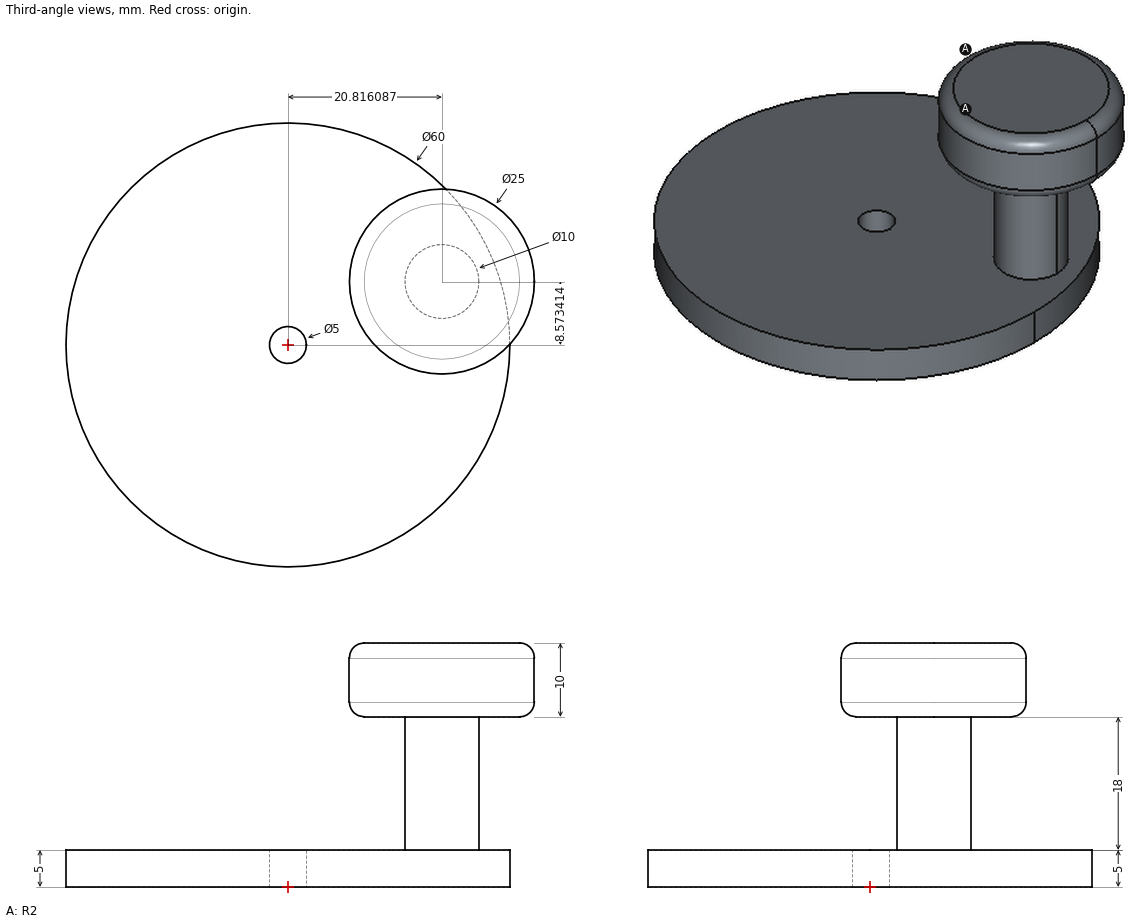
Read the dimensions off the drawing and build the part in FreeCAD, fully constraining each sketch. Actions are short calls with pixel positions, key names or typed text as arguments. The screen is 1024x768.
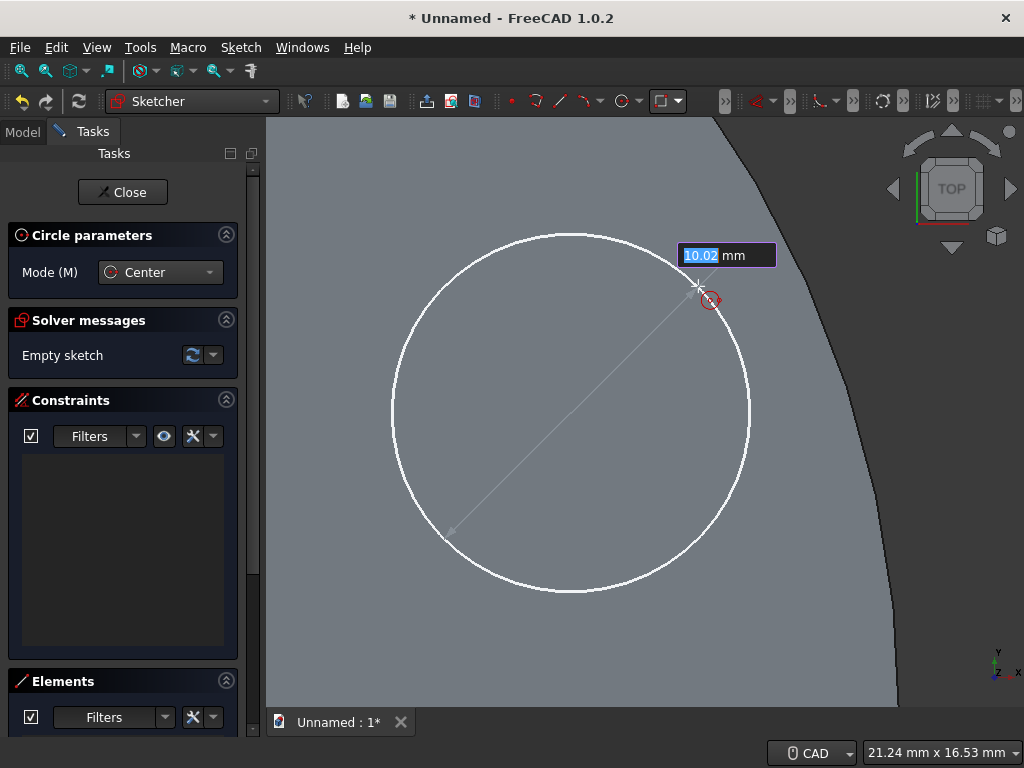
text(10)
key(Return)
key(Escape)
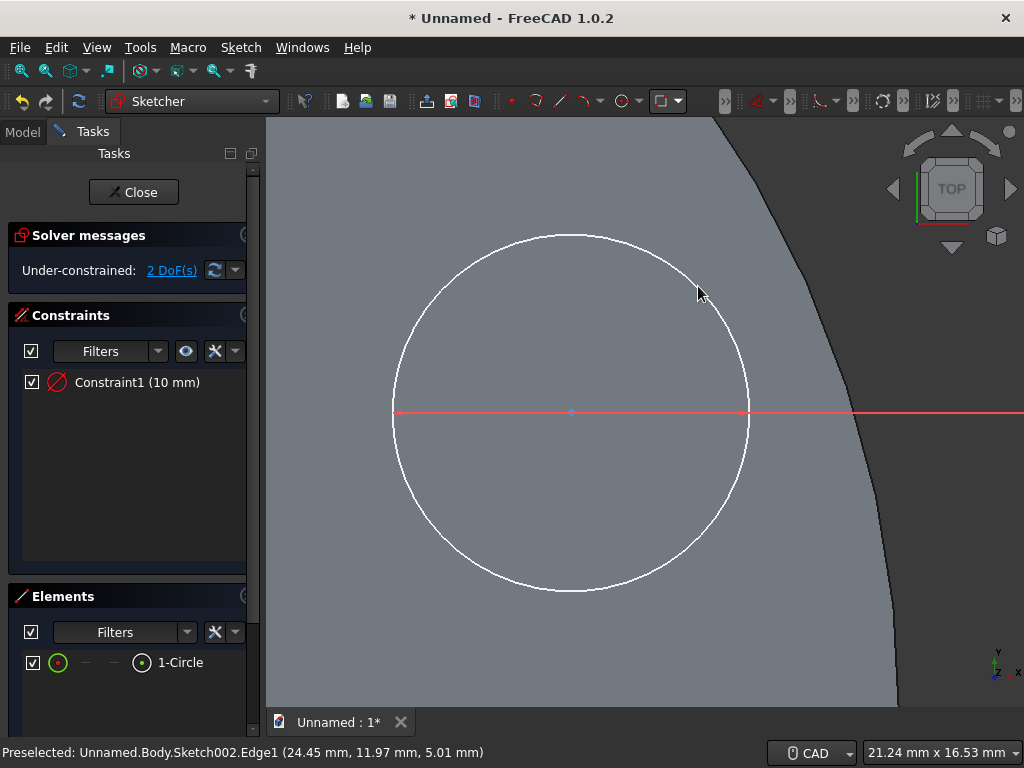
click(756, 102)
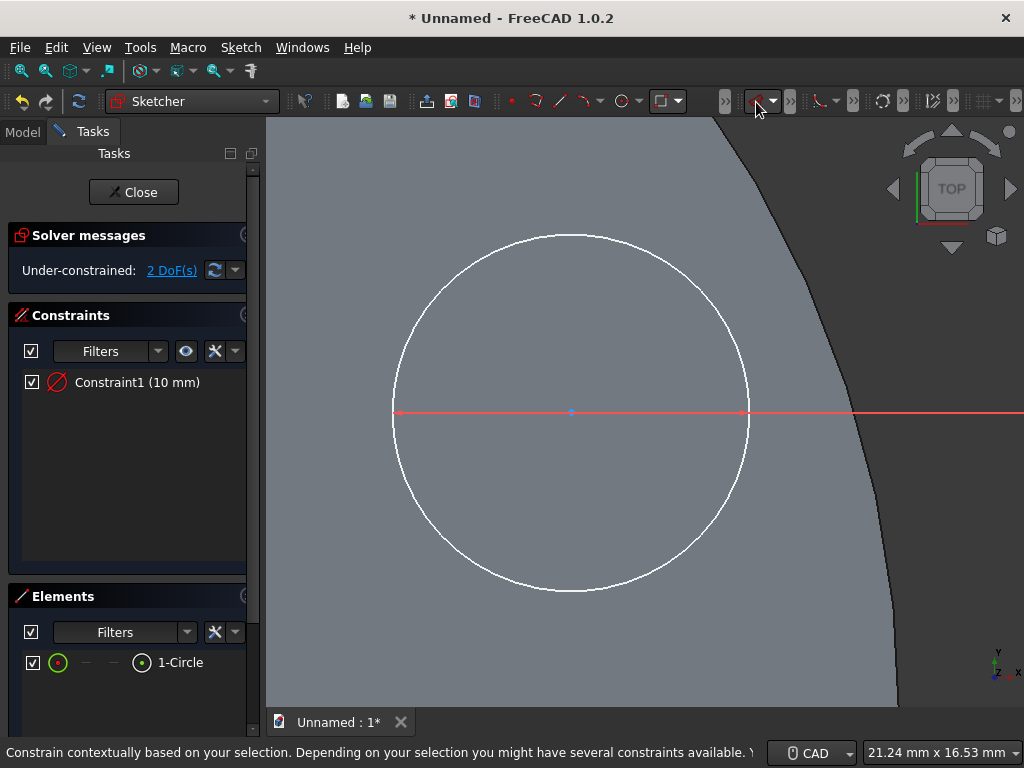
click(571, 413)
click(605, 546)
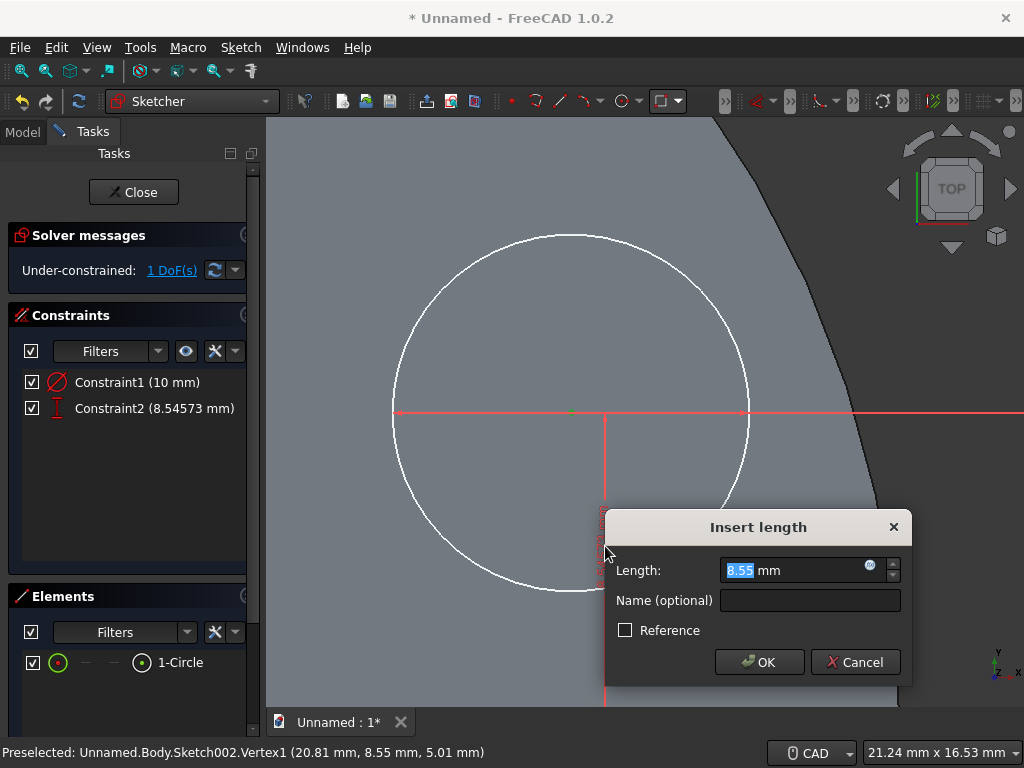
text(8.573414)
key(Return)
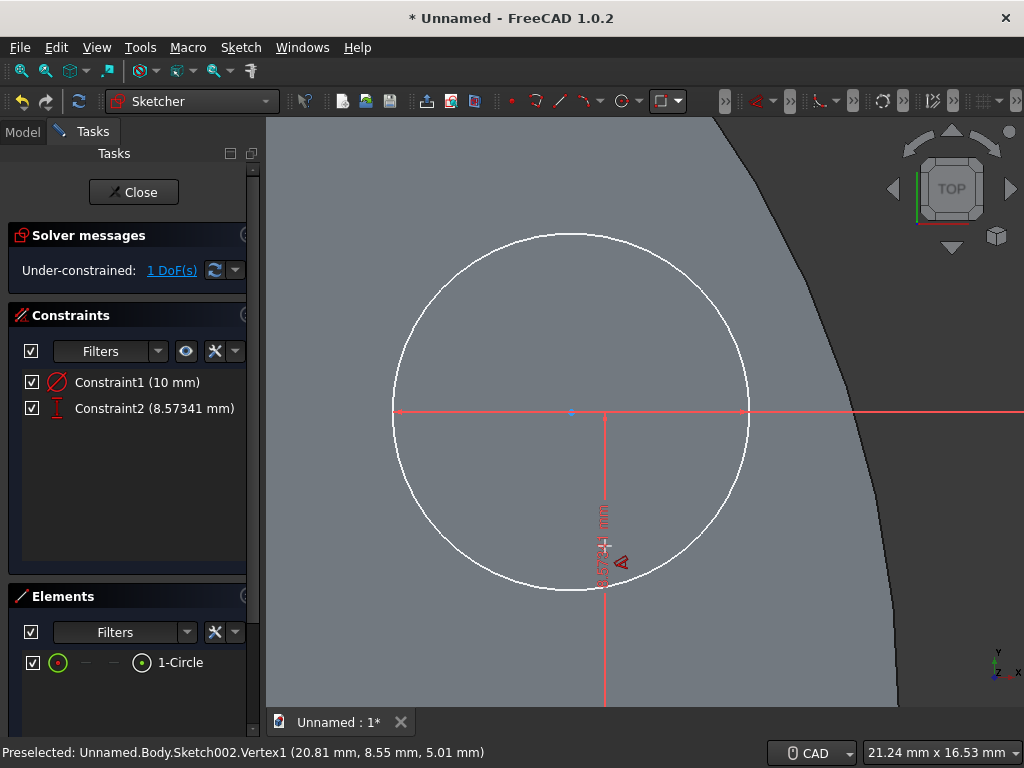
click(571, 412)
click(433, 378)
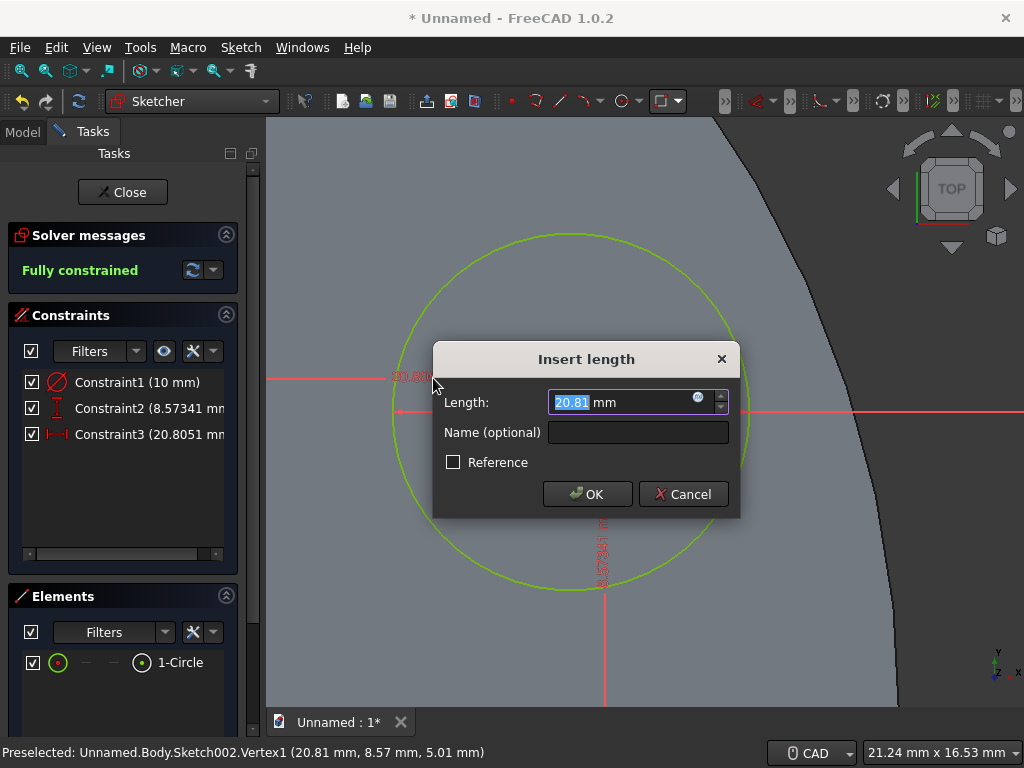
text(20.816087)
key(Return)
key(Escape)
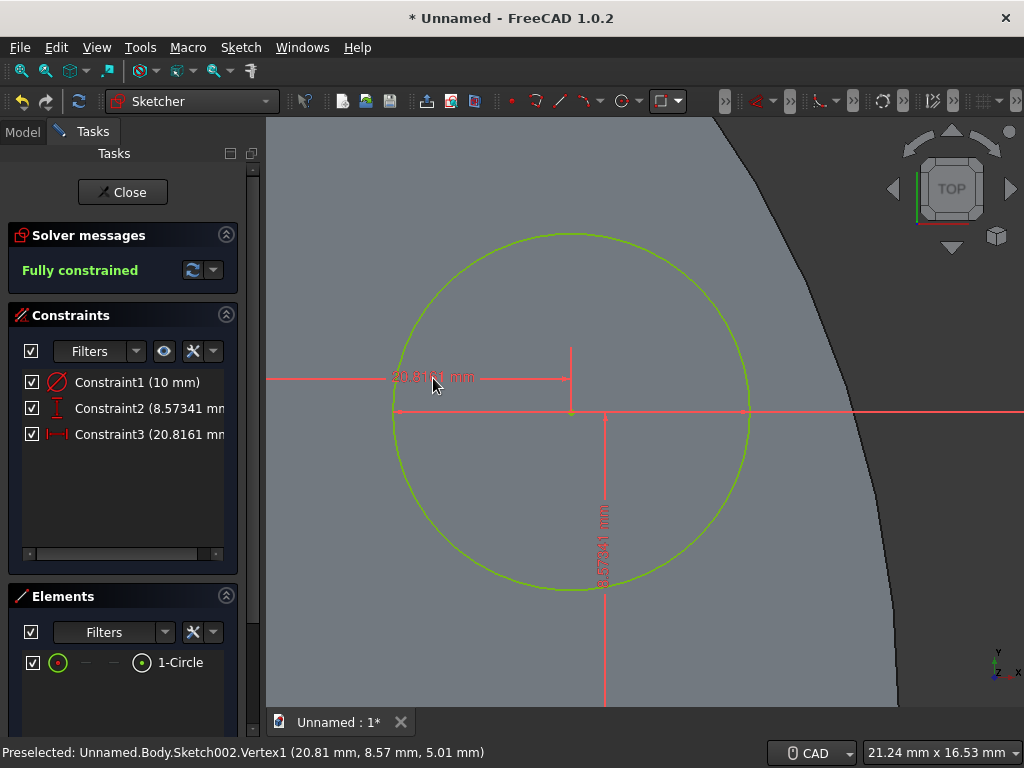
click(123, 192)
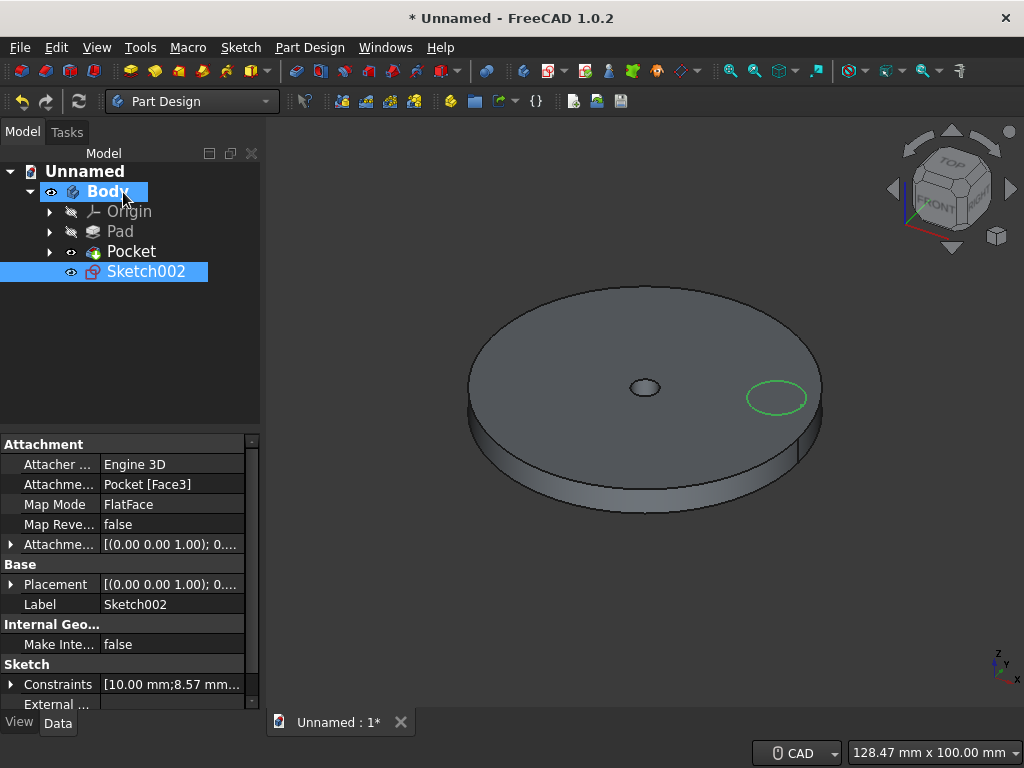
click(132, 72)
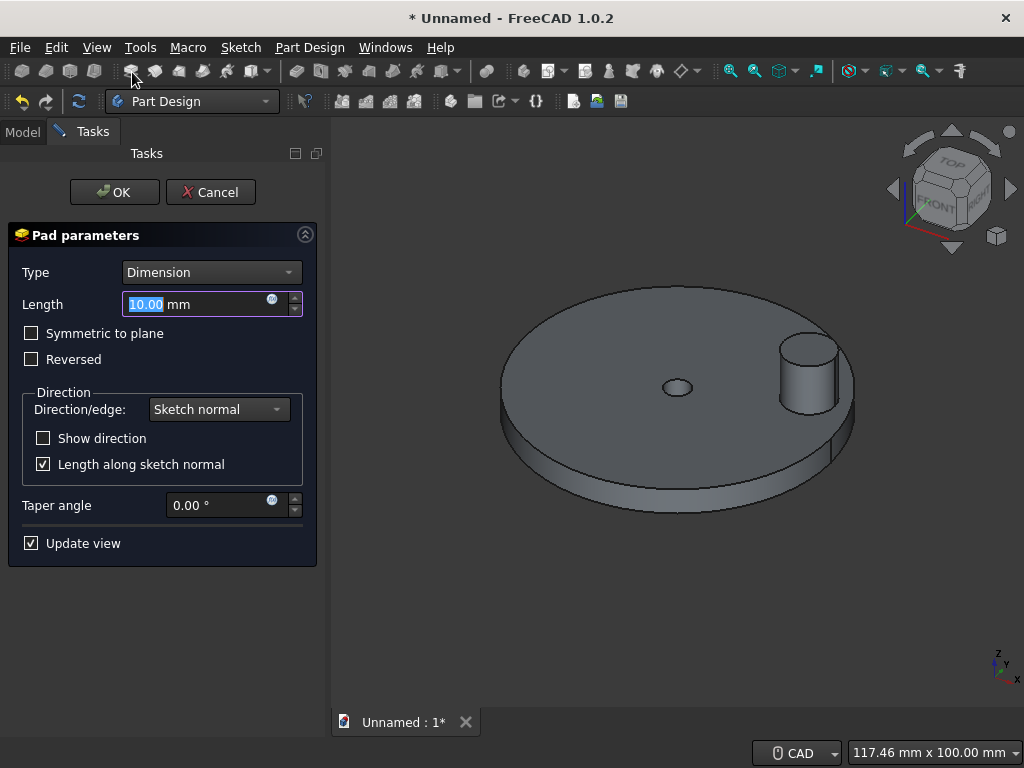
text(18)
key(Tab)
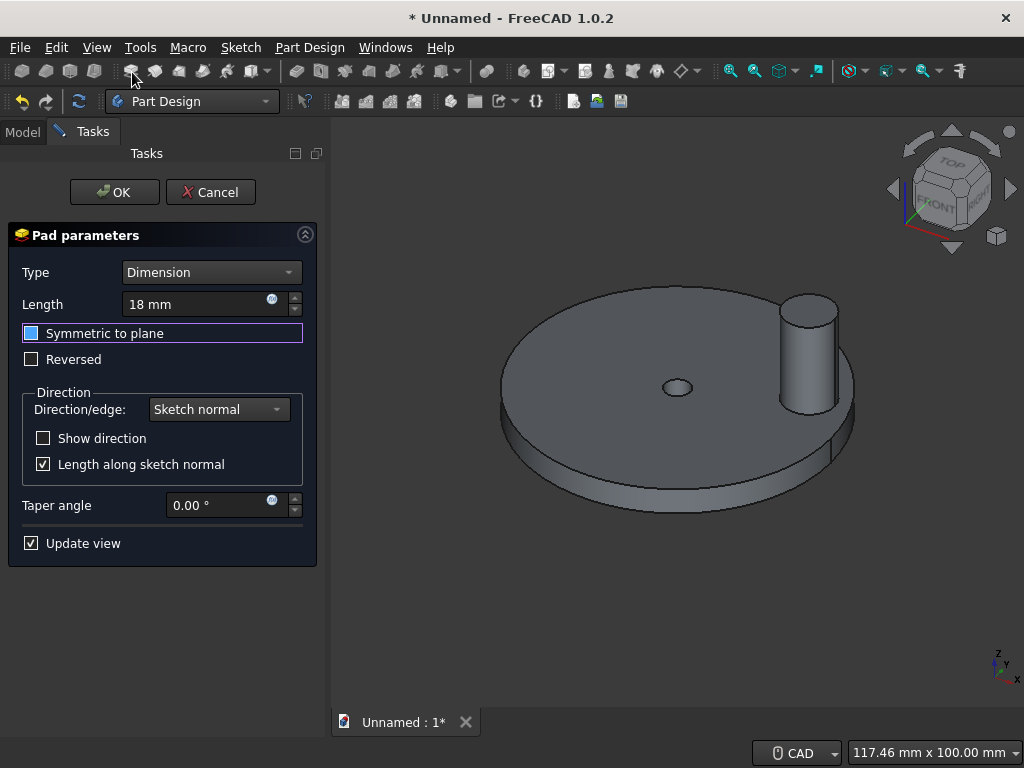
click(115, 192)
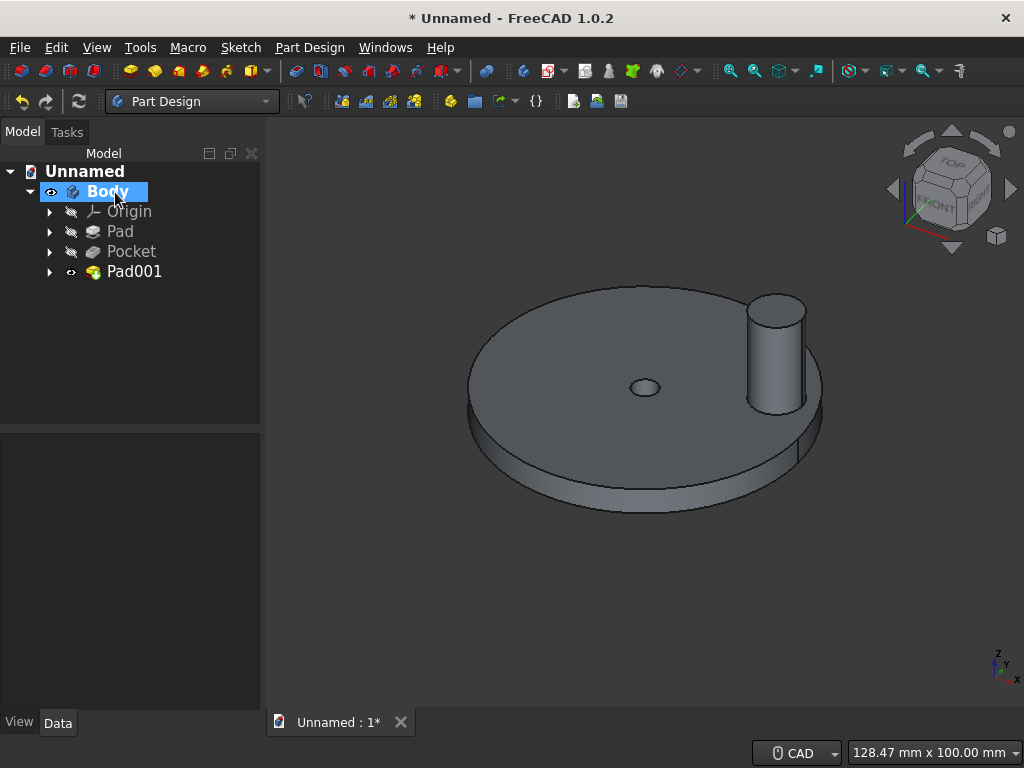
click(777, 310)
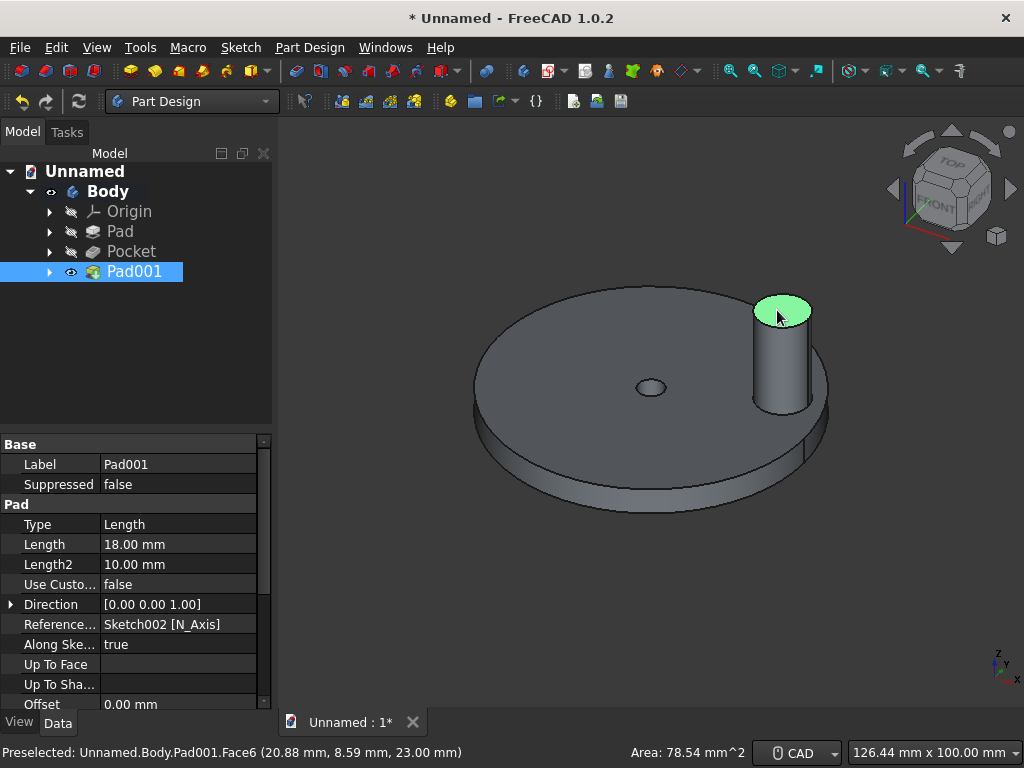
click(548, 72)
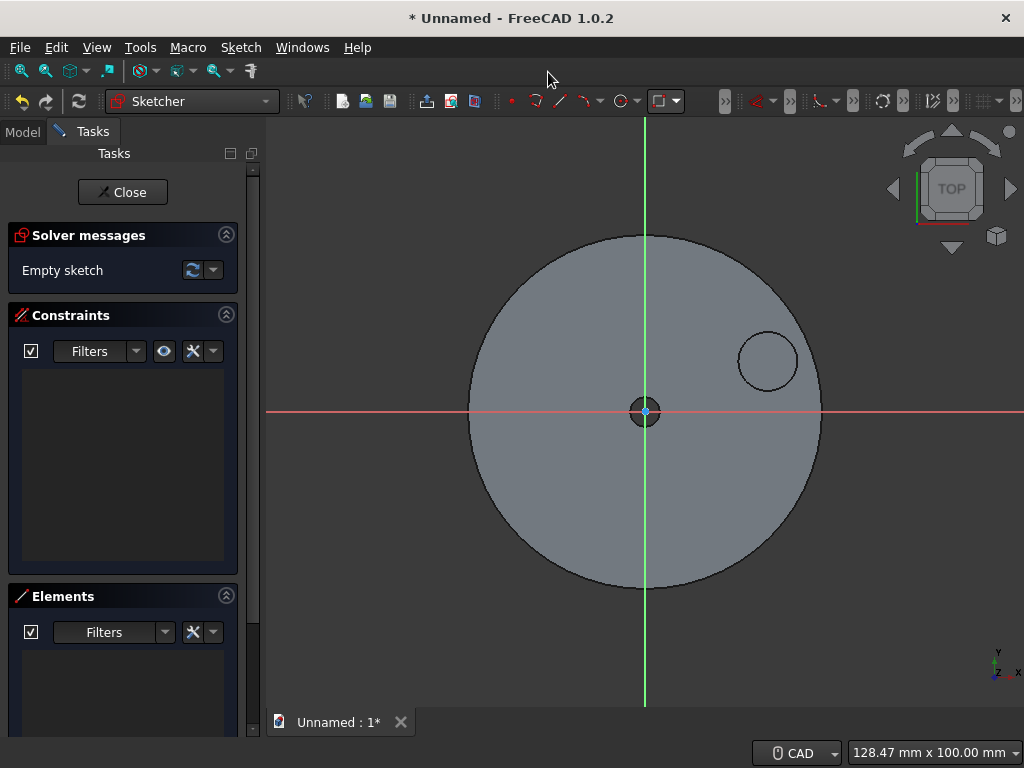
scroll(859, 320, up, 4)